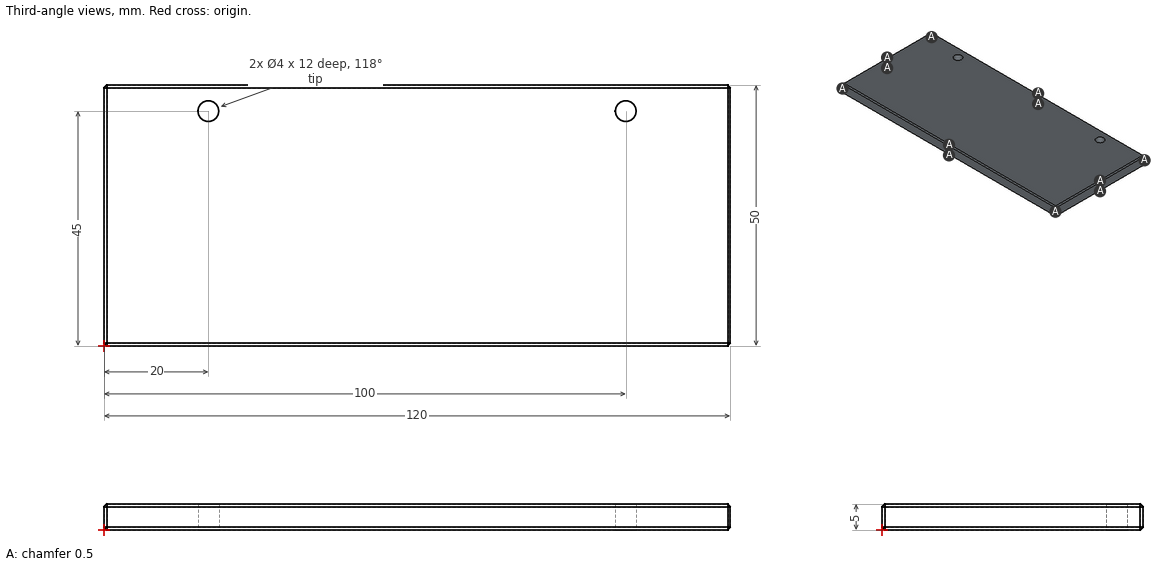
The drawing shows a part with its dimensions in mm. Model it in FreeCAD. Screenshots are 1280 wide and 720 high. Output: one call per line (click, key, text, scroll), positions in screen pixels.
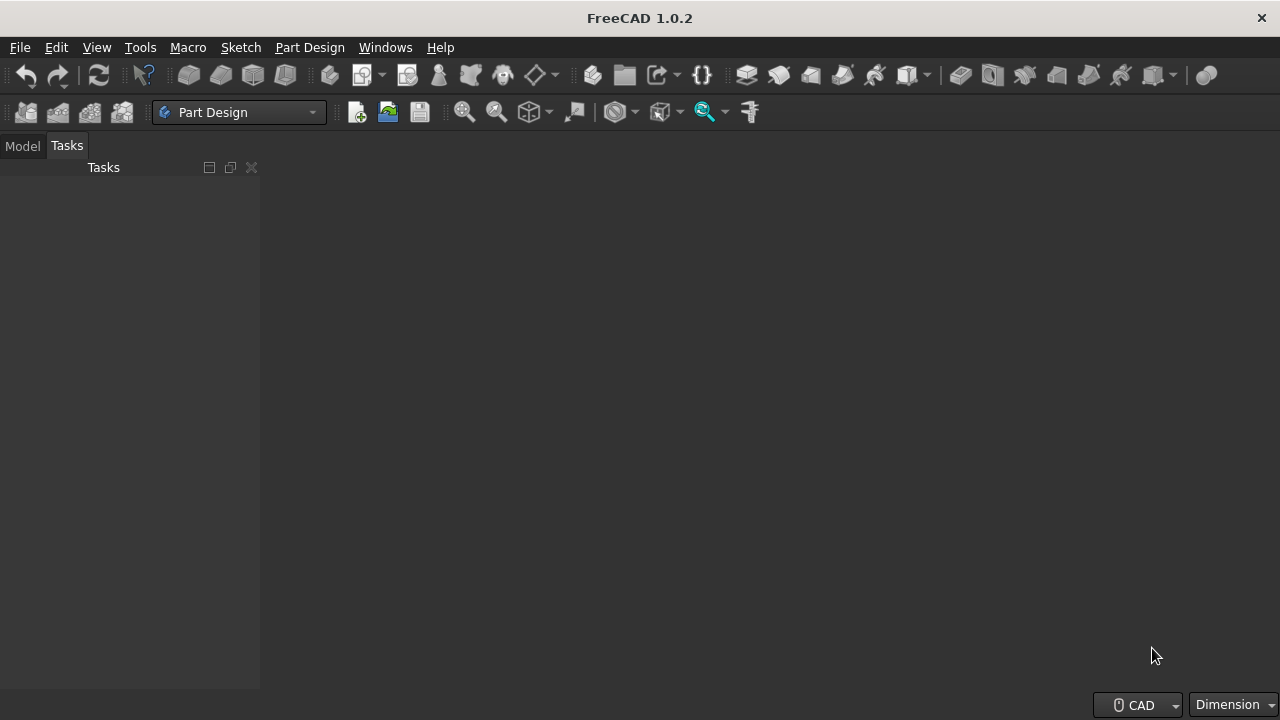
click(356, 112)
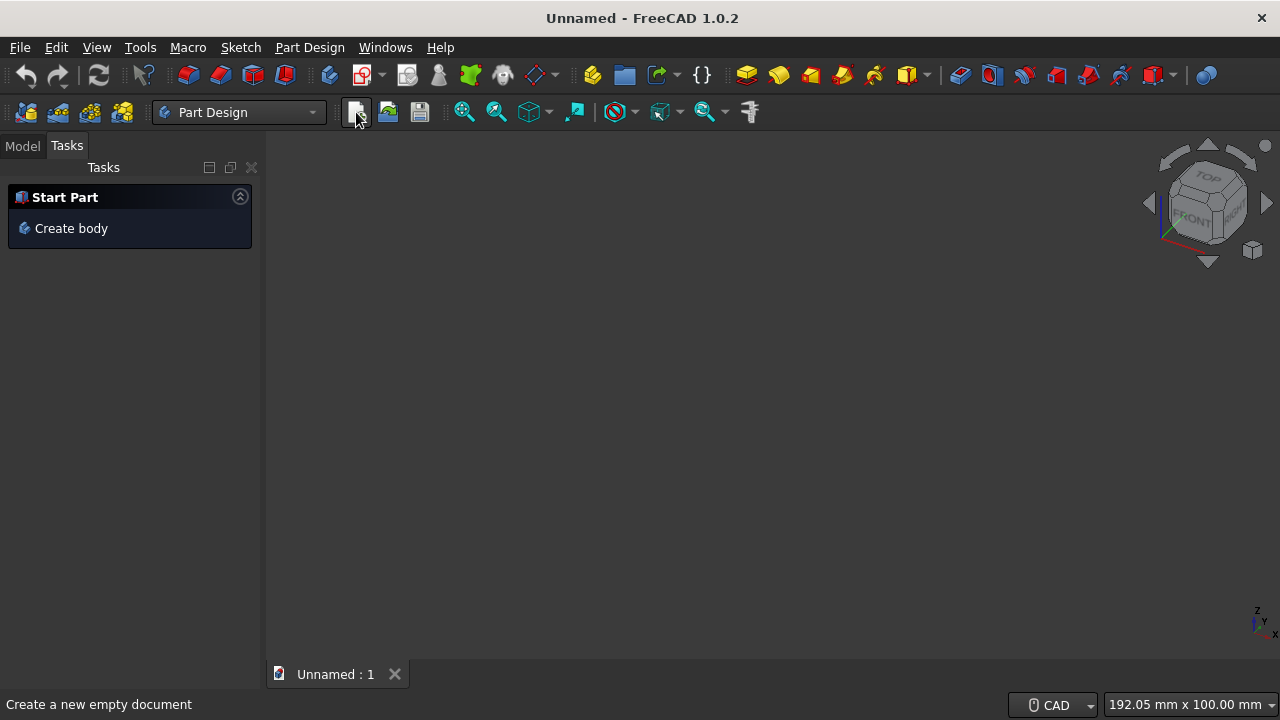
click(362, 76)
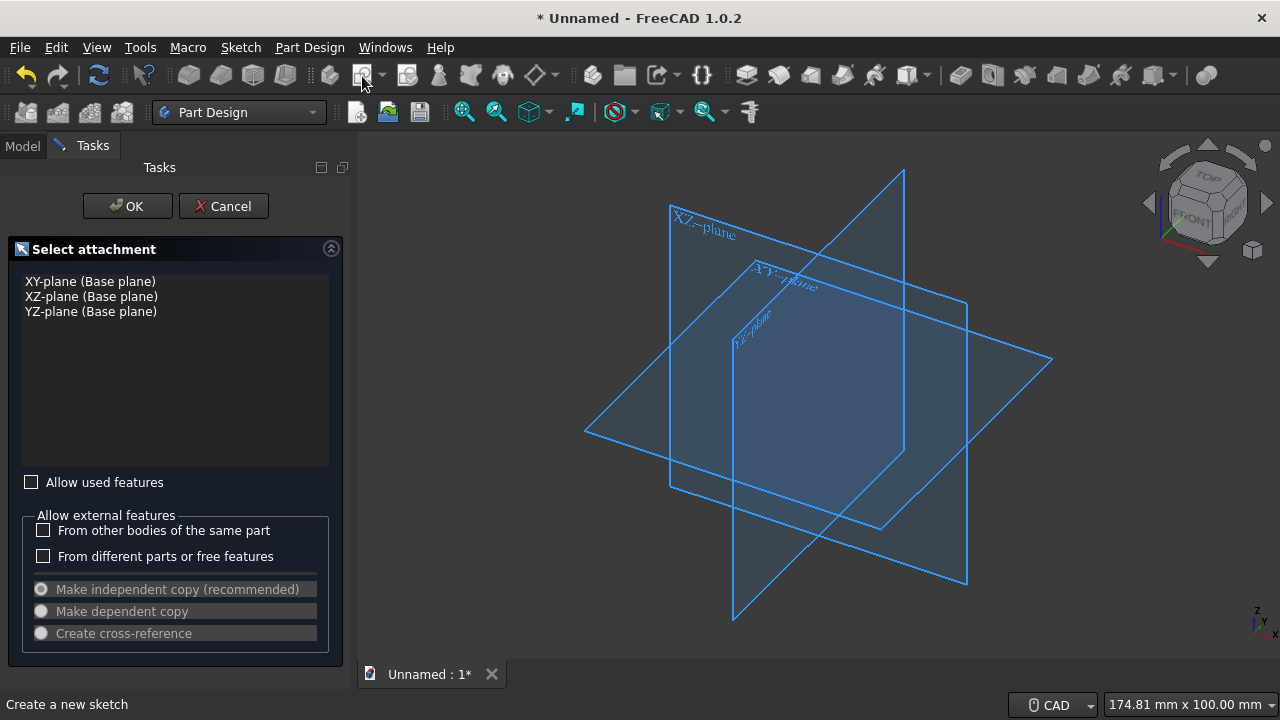
click(82, 282)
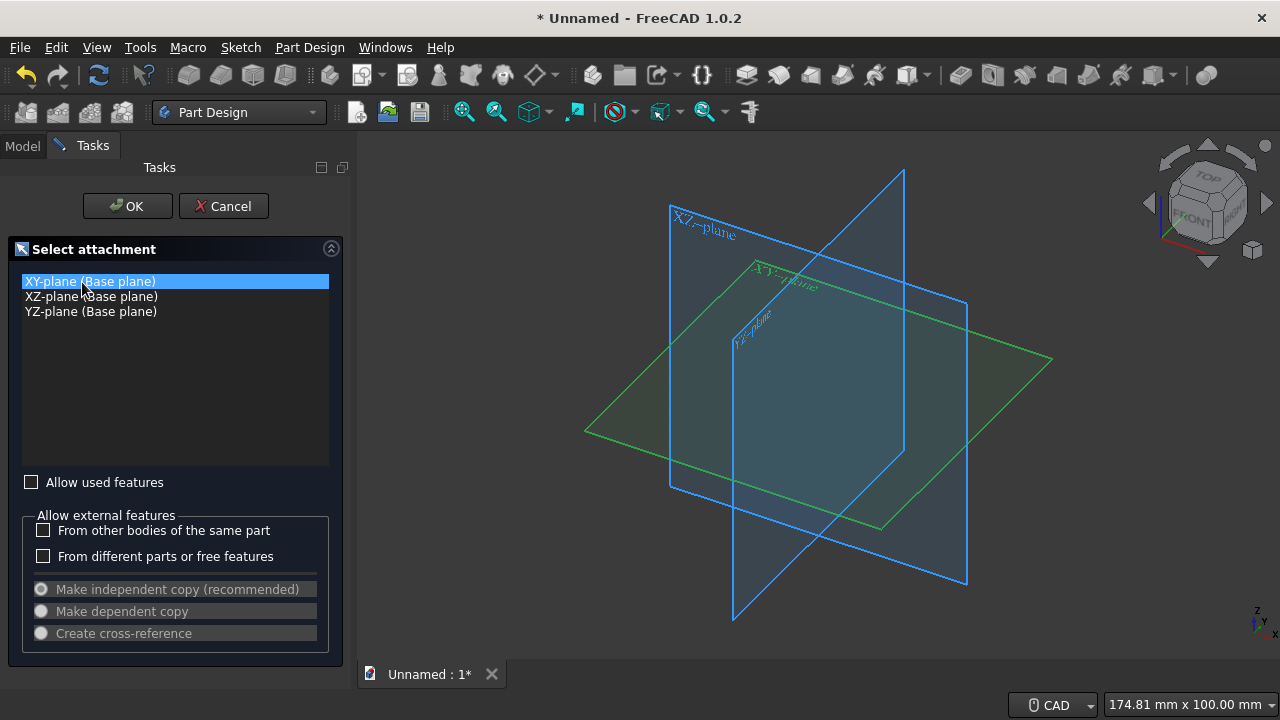
click(128, 206)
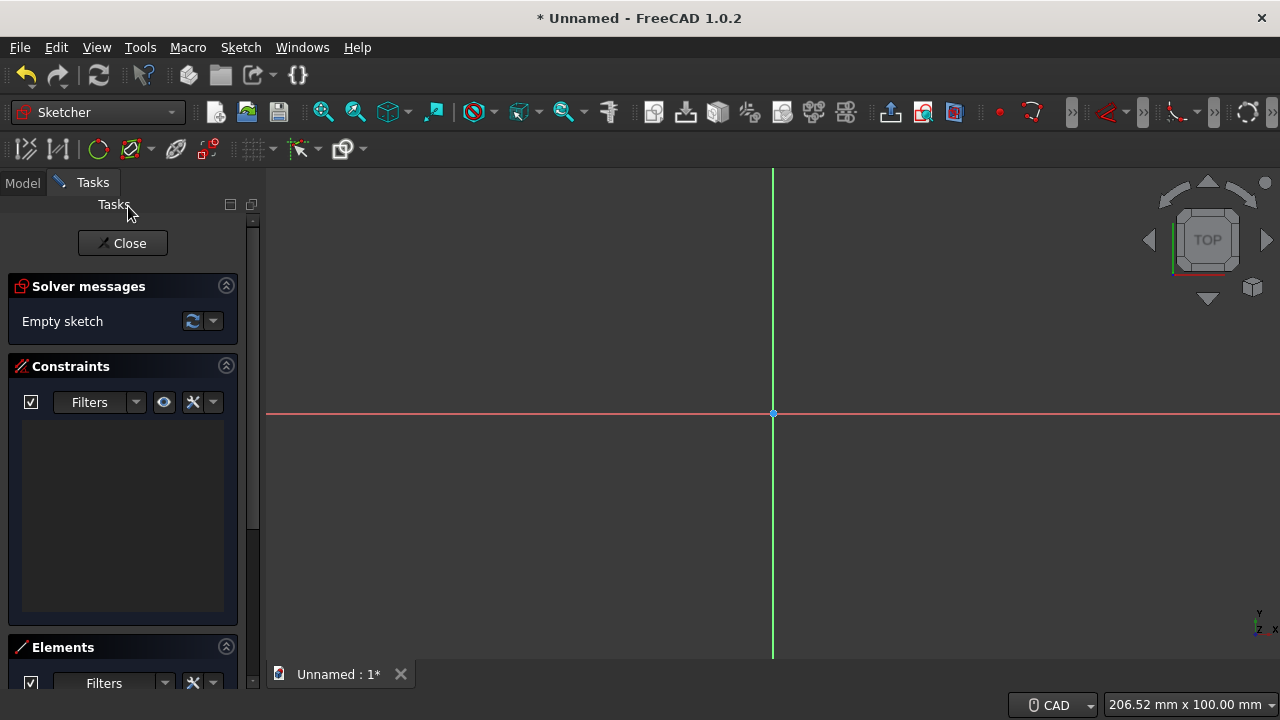
scroll(294, 631, down, 2)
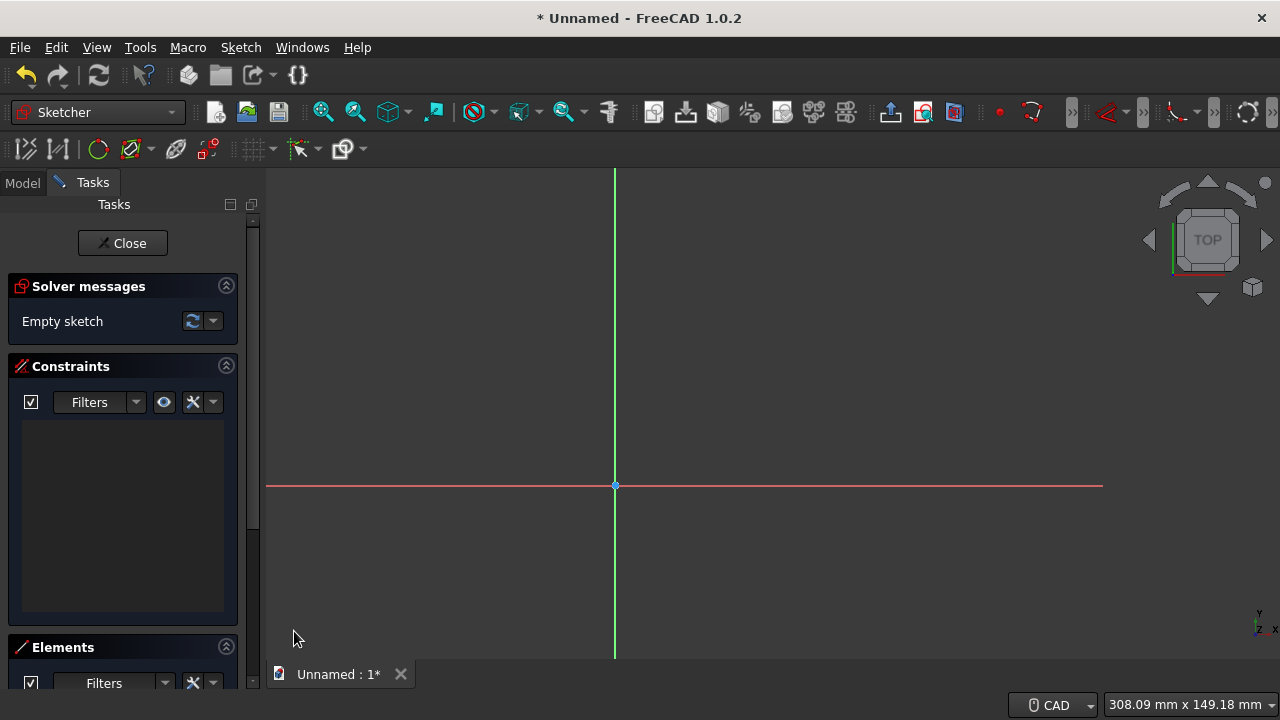
scroll(1032, 382, up, 2)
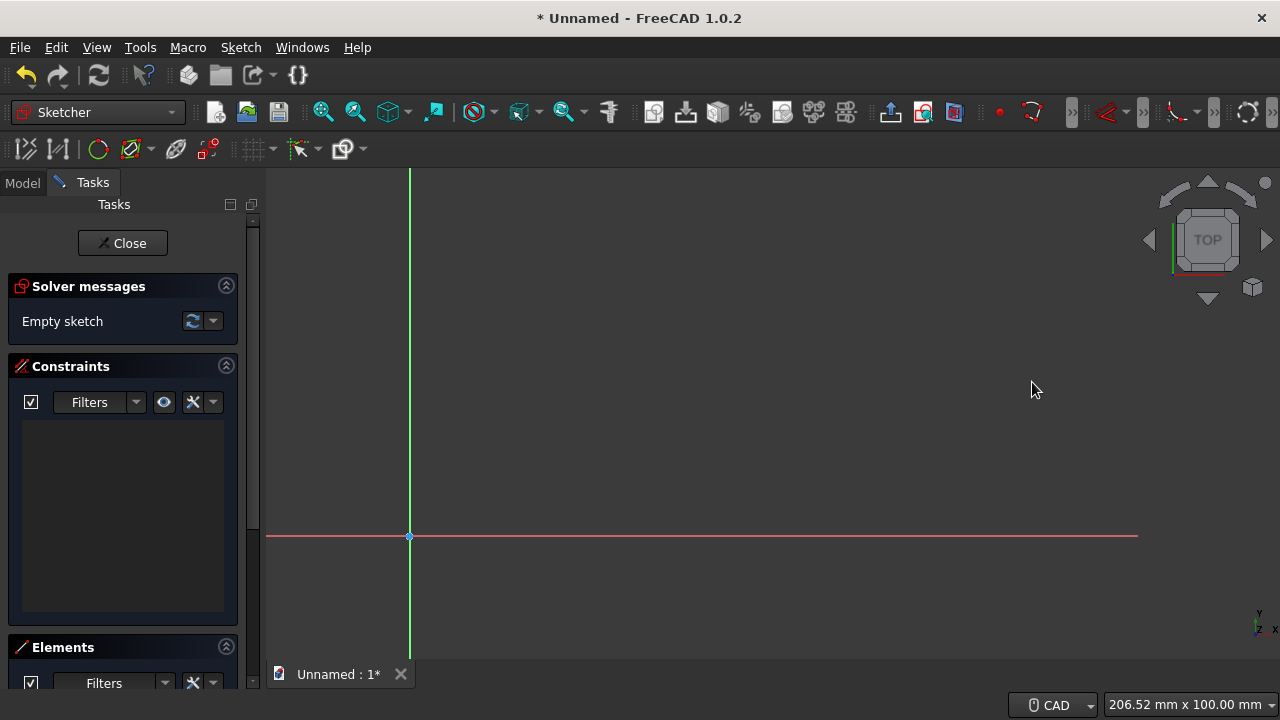
key(g)
key(r)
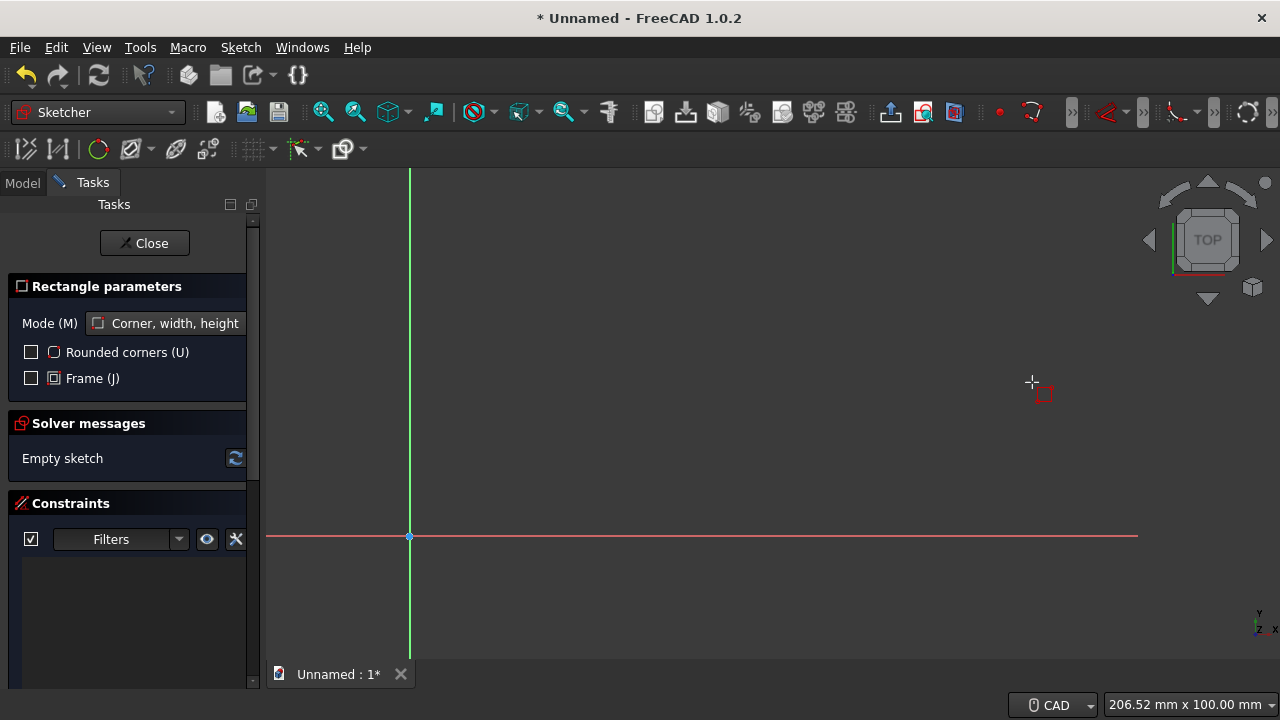
click(410, 536)
move(999, 291)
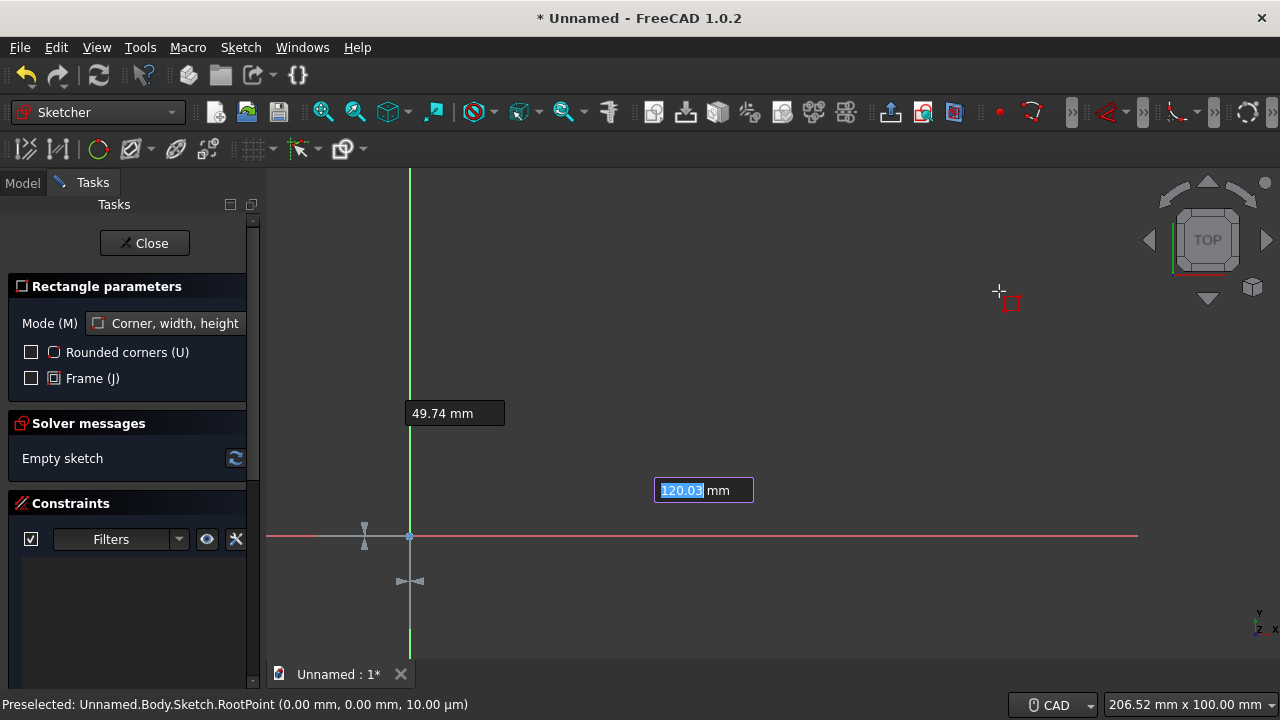
text(120)
key(Tab)
text(50)
key(Return)
key(Escape)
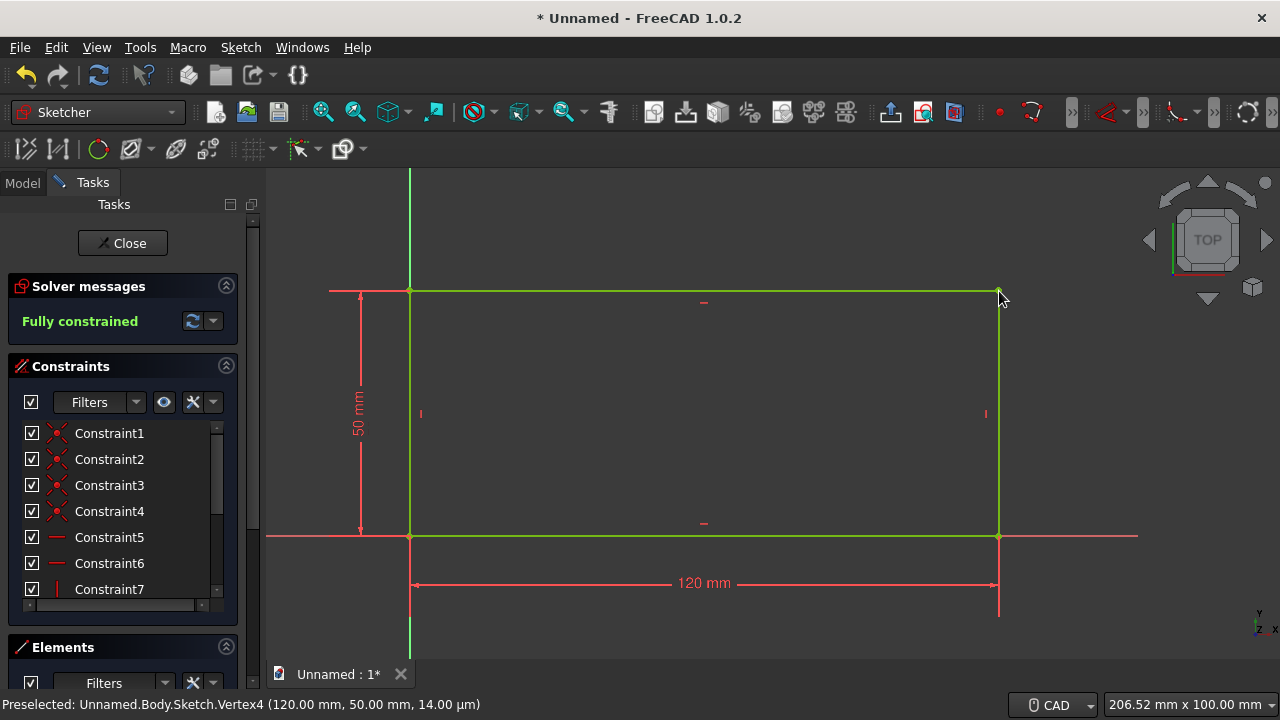
click(123, 243)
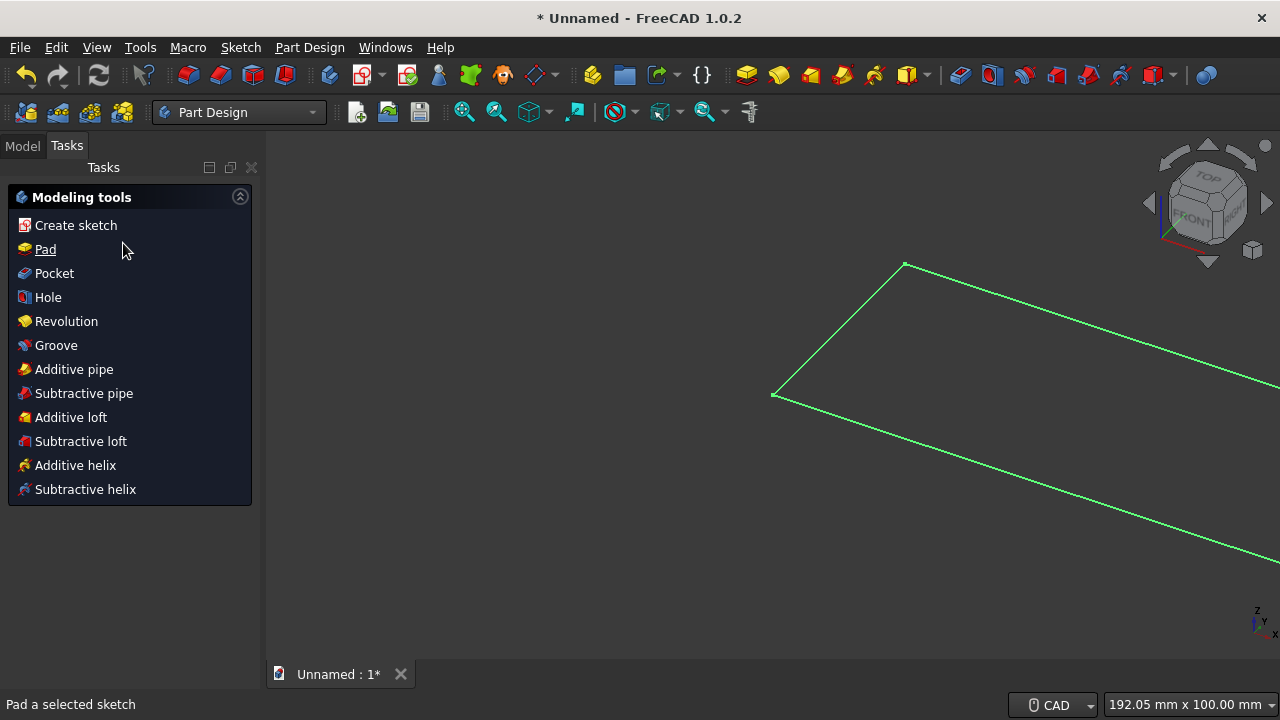
click(748, 76)